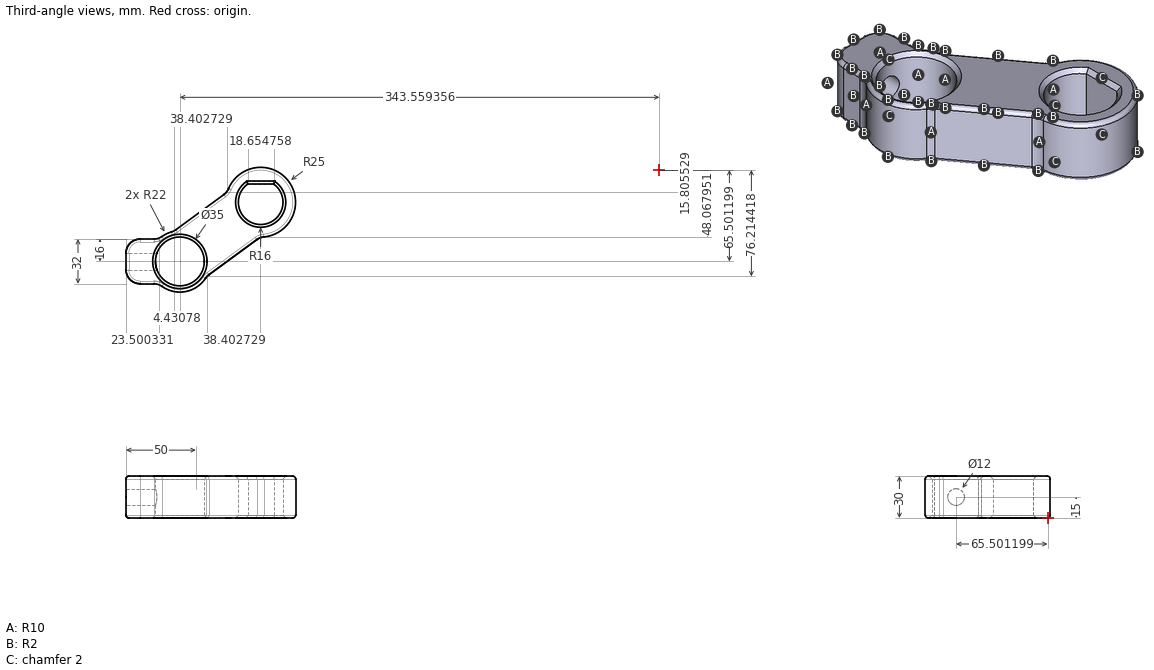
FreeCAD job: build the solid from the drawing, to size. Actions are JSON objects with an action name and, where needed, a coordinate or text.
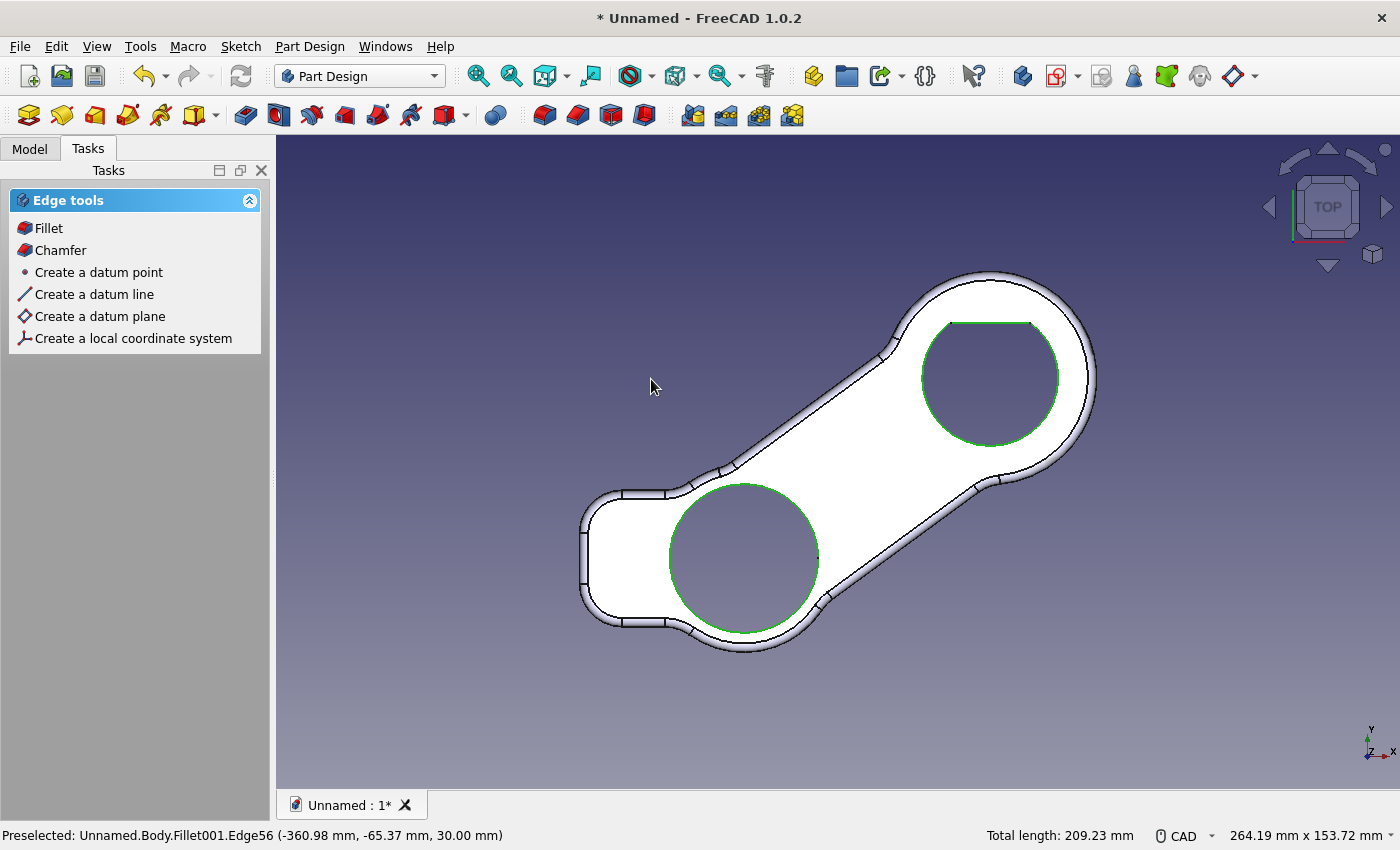
{"action": "key", "text": "1"}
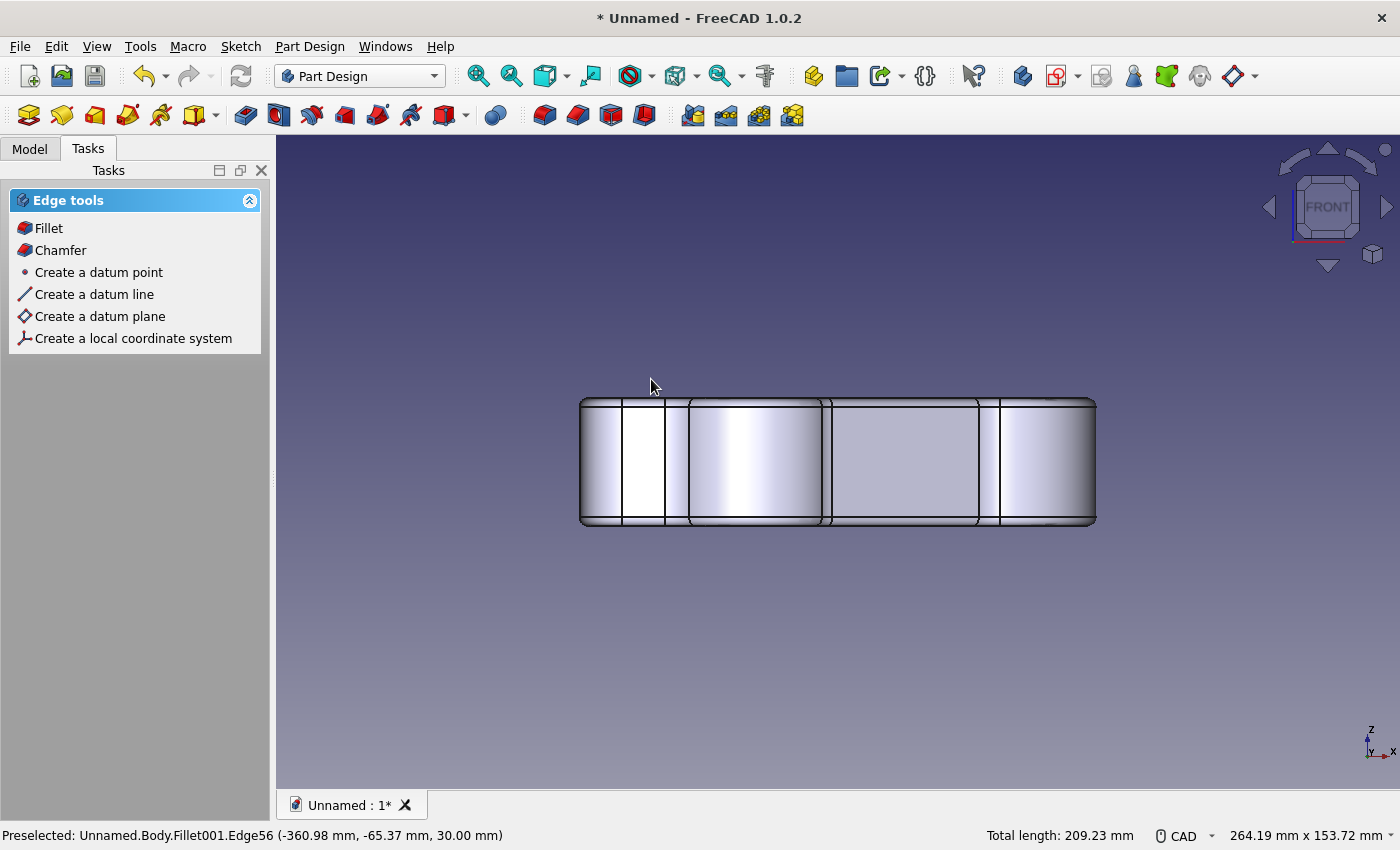
{"action": "key", "text": "3"}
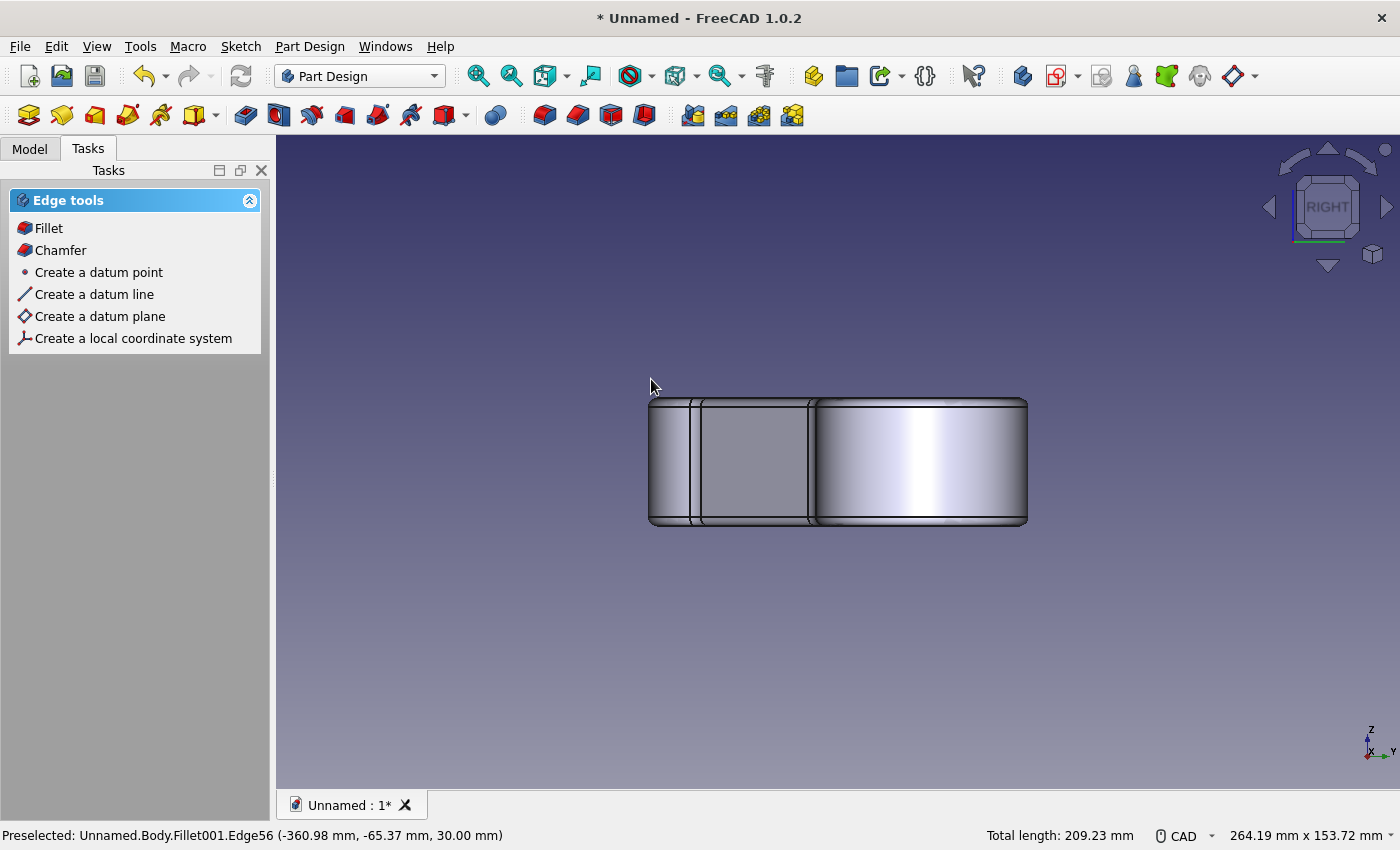
{"action": "left_click", "coordinate": [479, 76]}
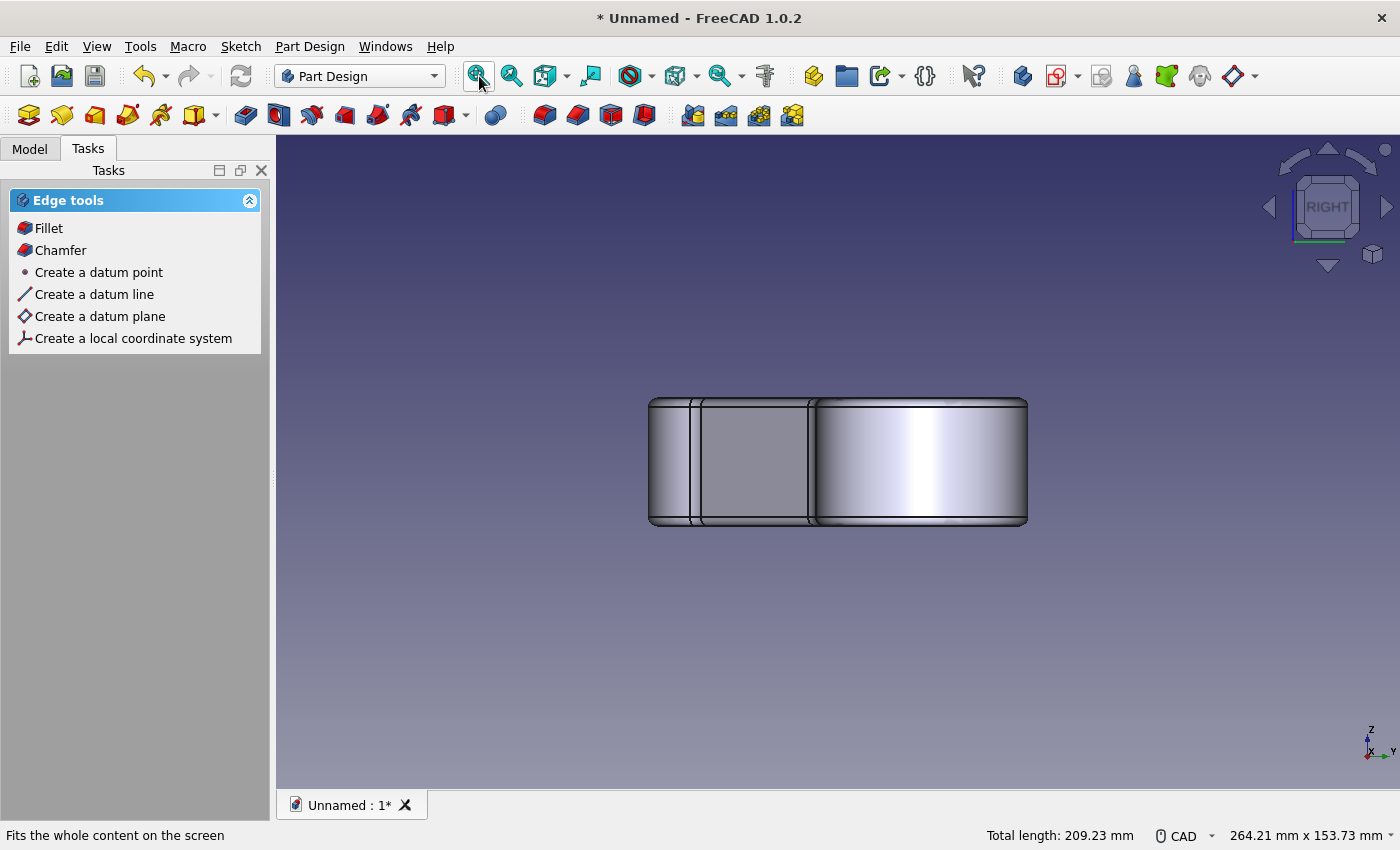
{"action": "key", "text": "5"}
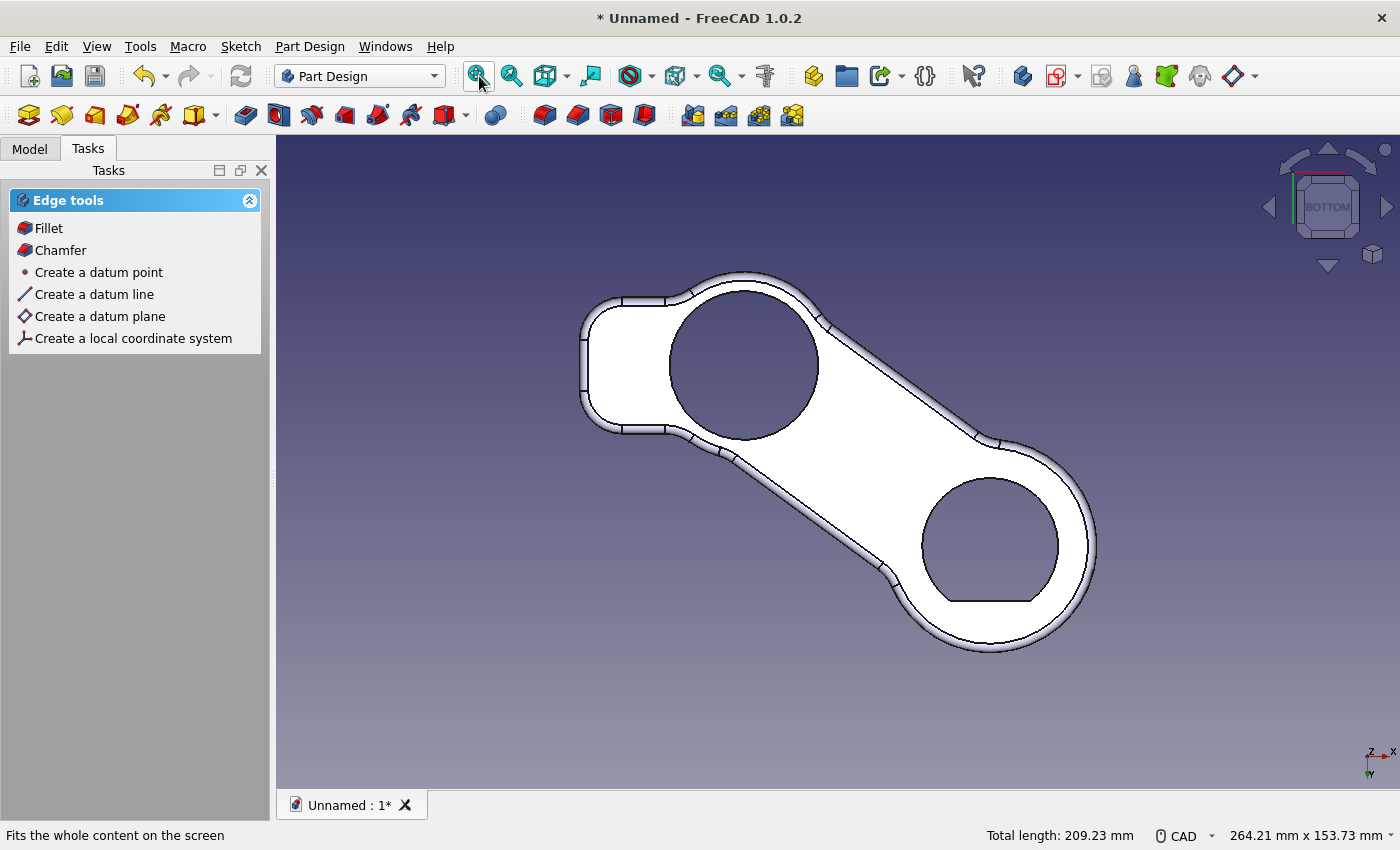
{"action": "left_click", "coordinate": [990, 477], "text": "ctrl"}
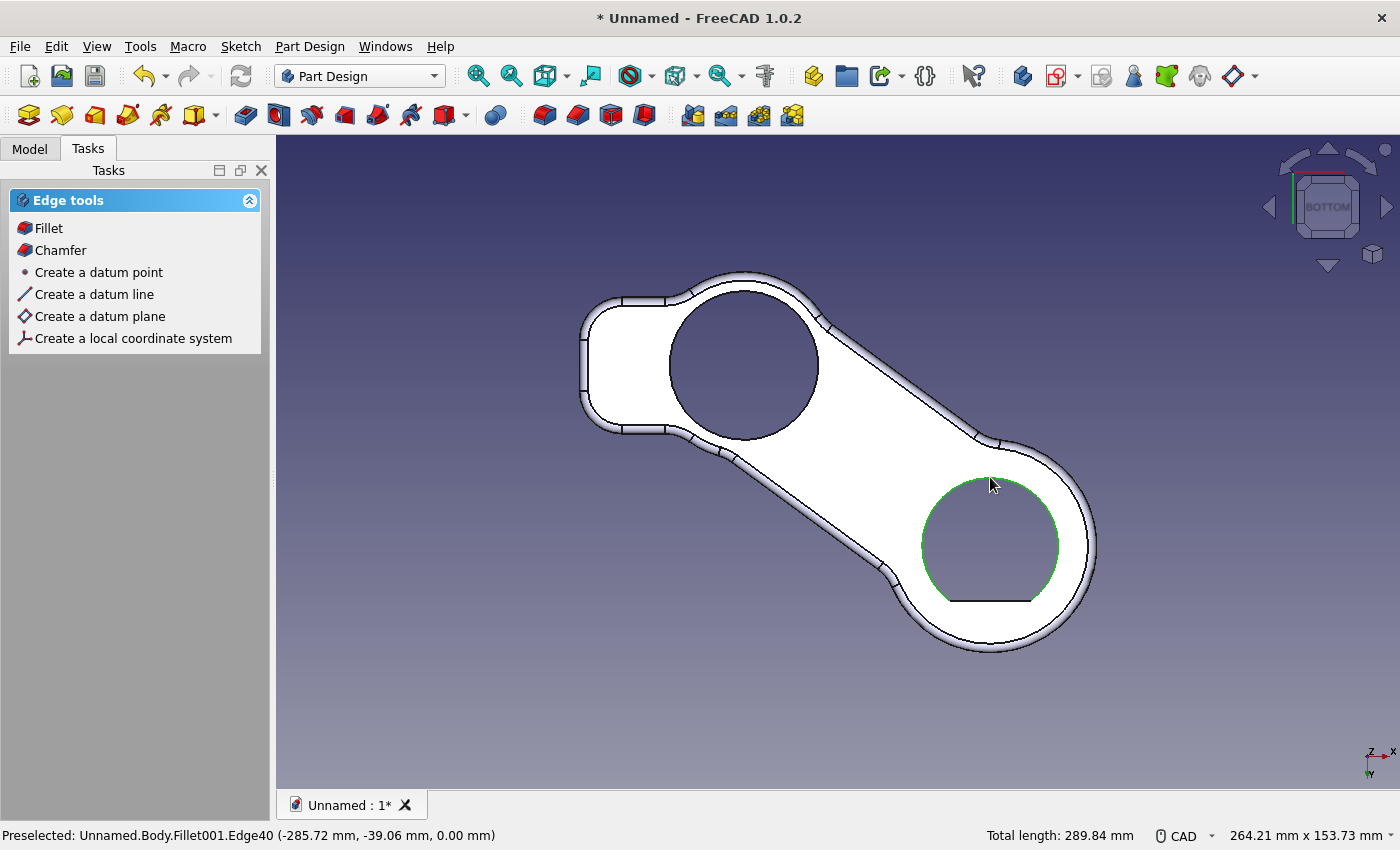
{"action": "left_click", "coordinate": [669, 364], "text": "ctrl"}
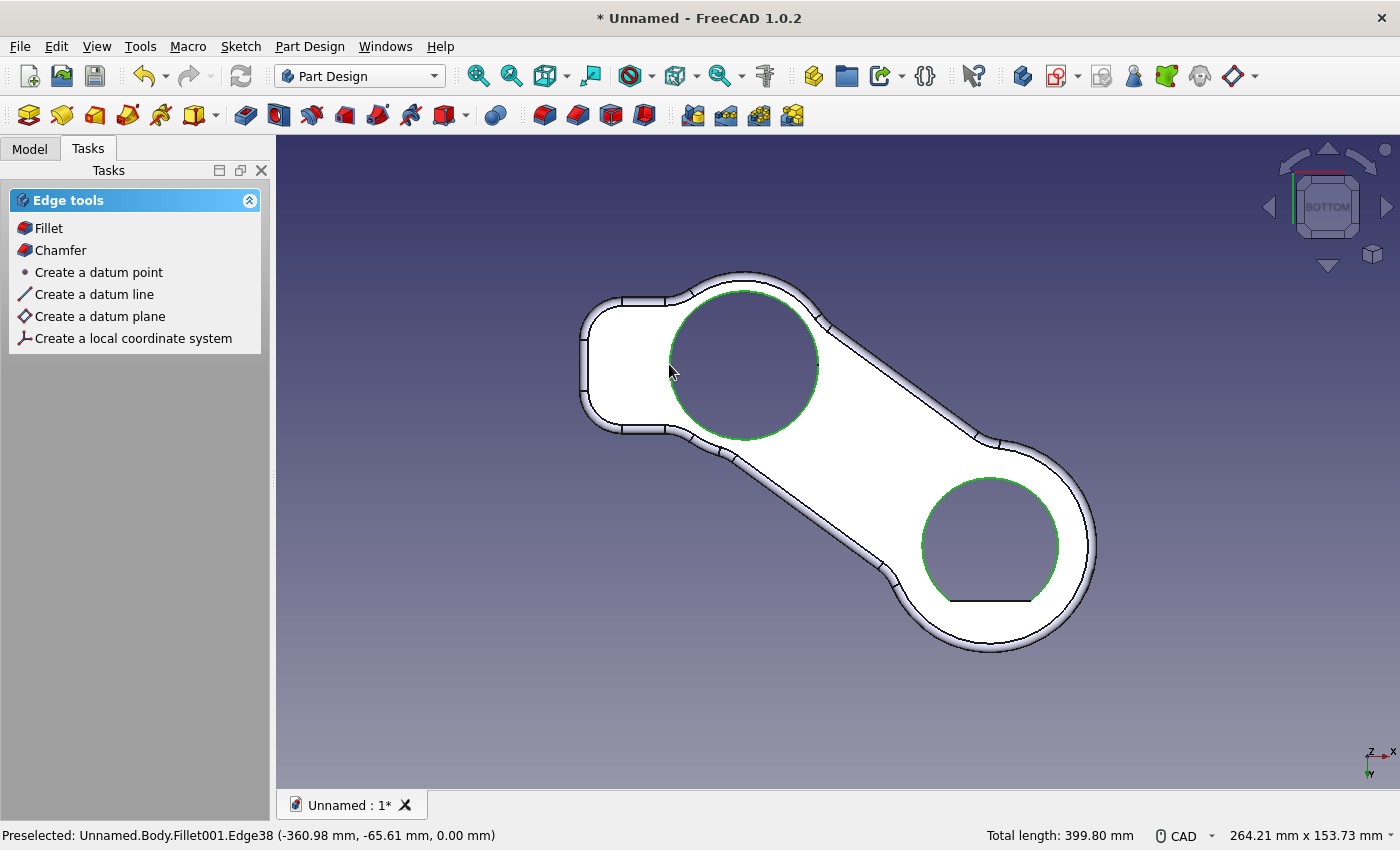
{"action": "key", "text": "4"}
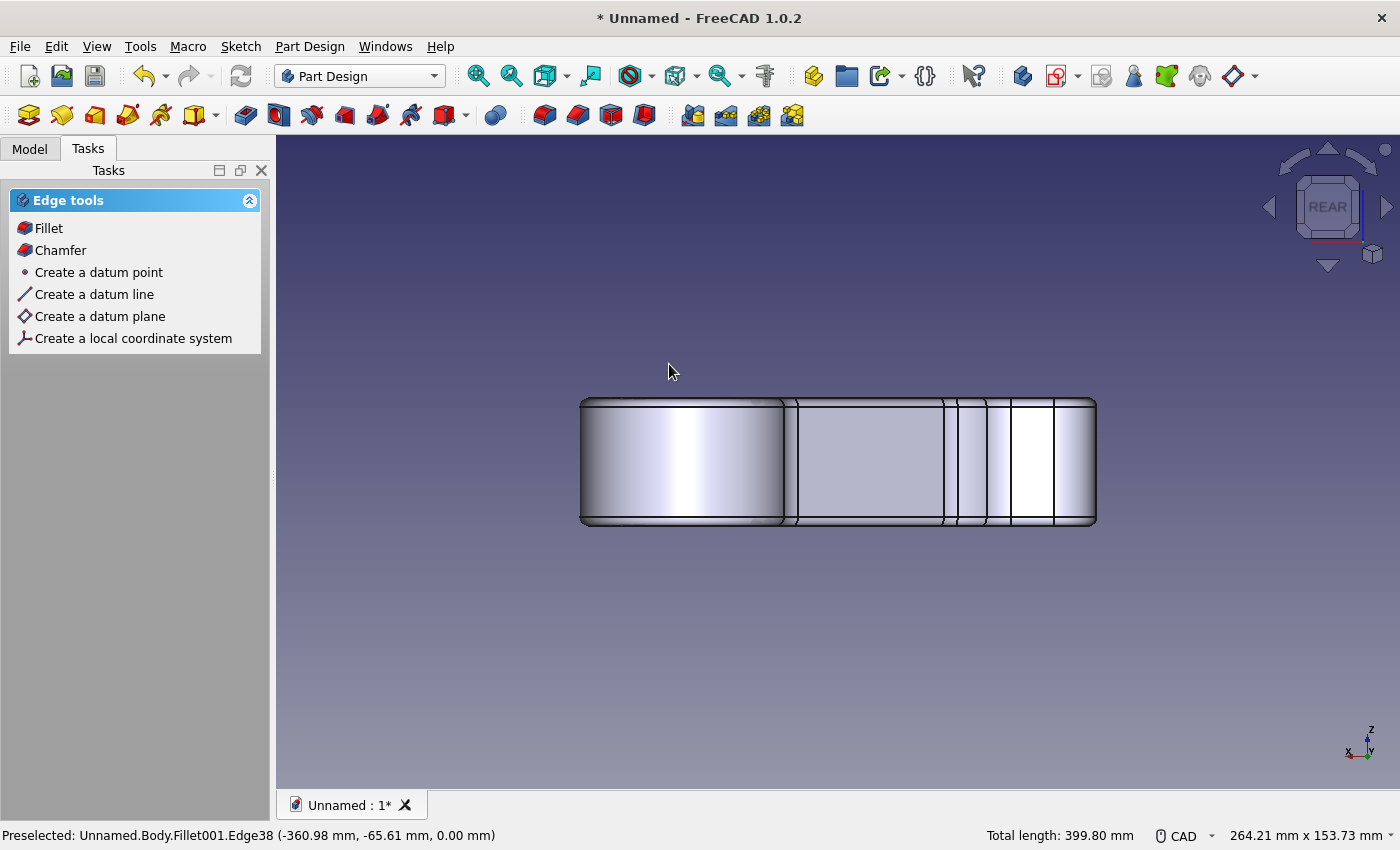
{"action": "key", "text": "6"}